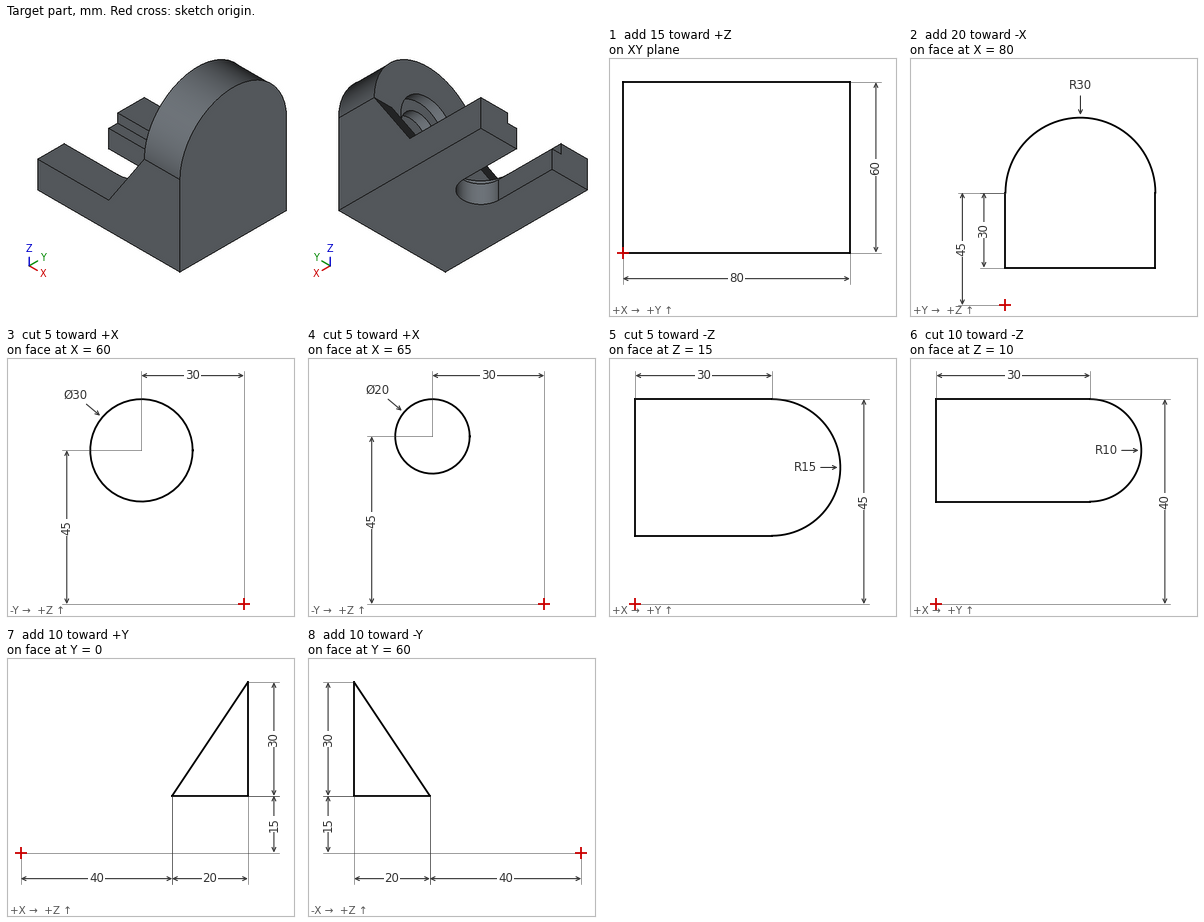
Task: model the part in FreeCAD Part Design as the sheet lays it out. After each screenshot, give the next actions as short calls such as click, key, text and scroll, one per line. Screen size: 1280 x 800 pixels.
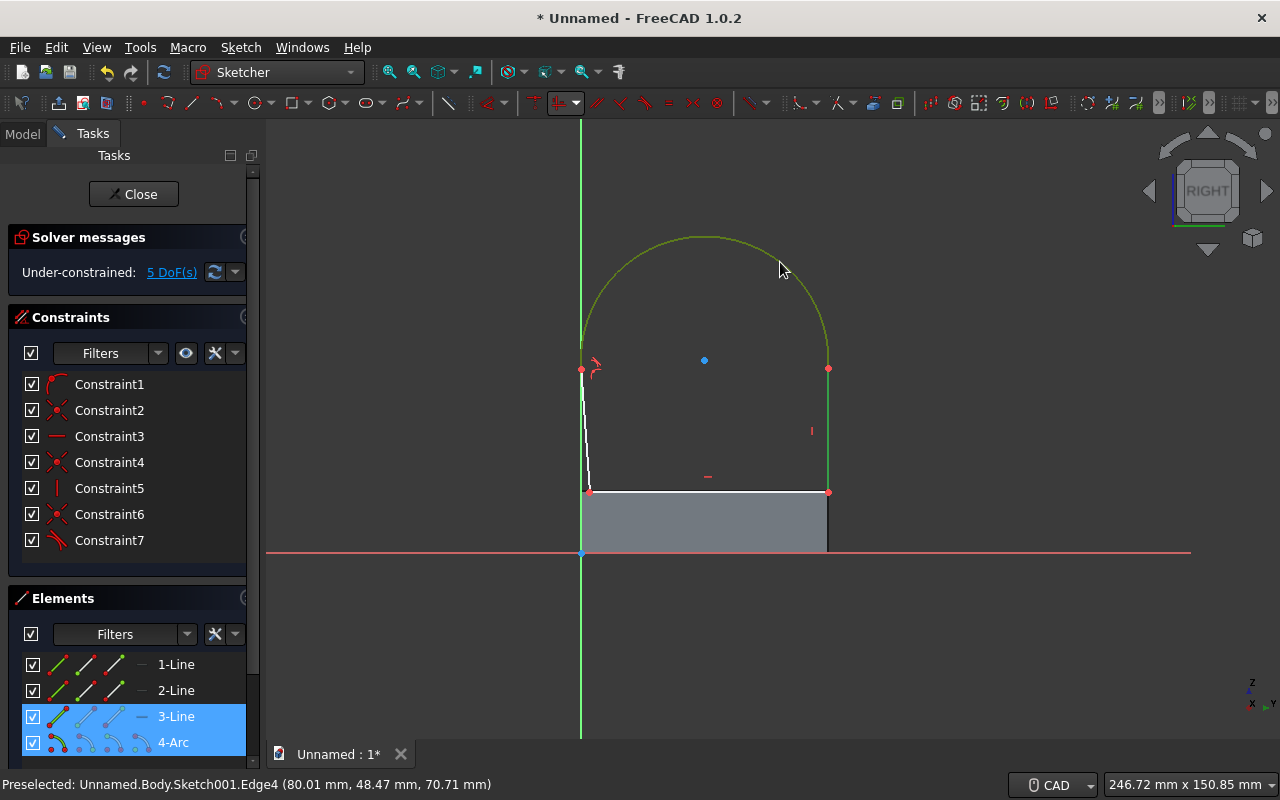
click(646, 104)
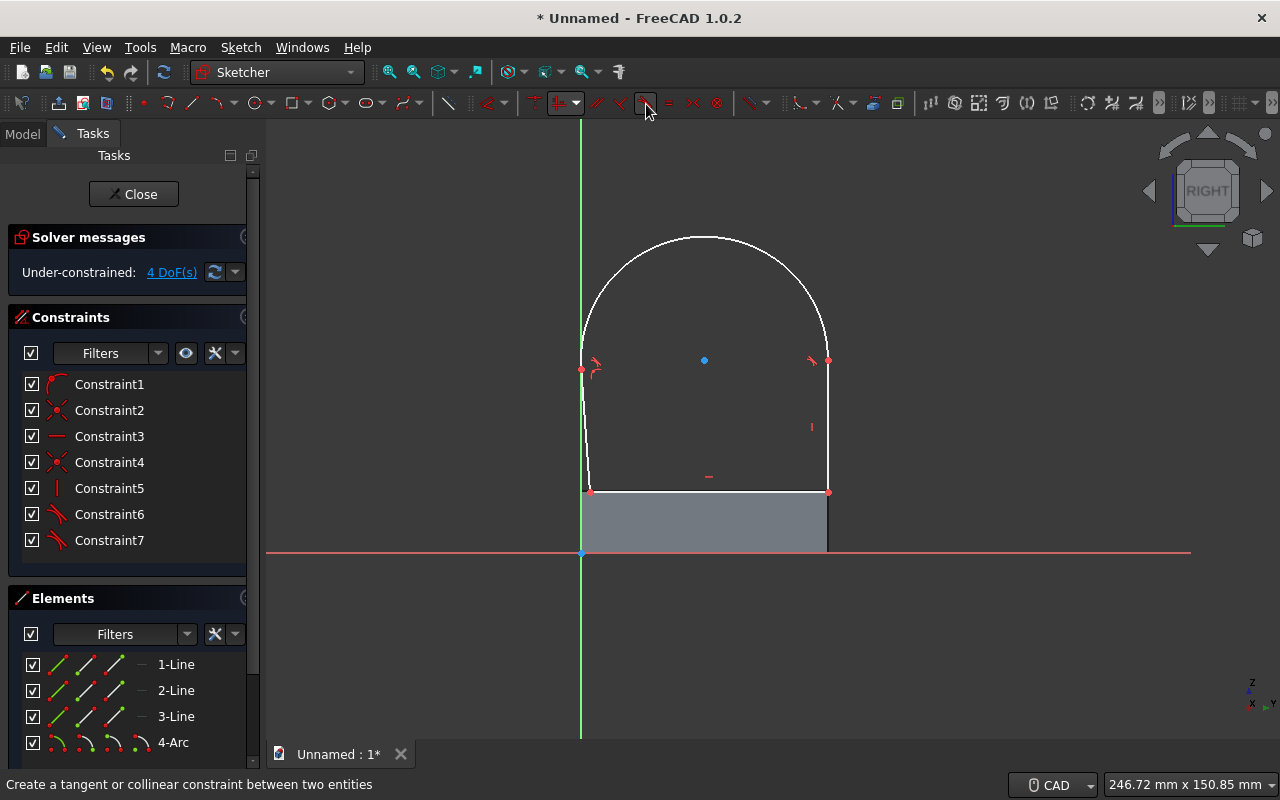
click(584, 406)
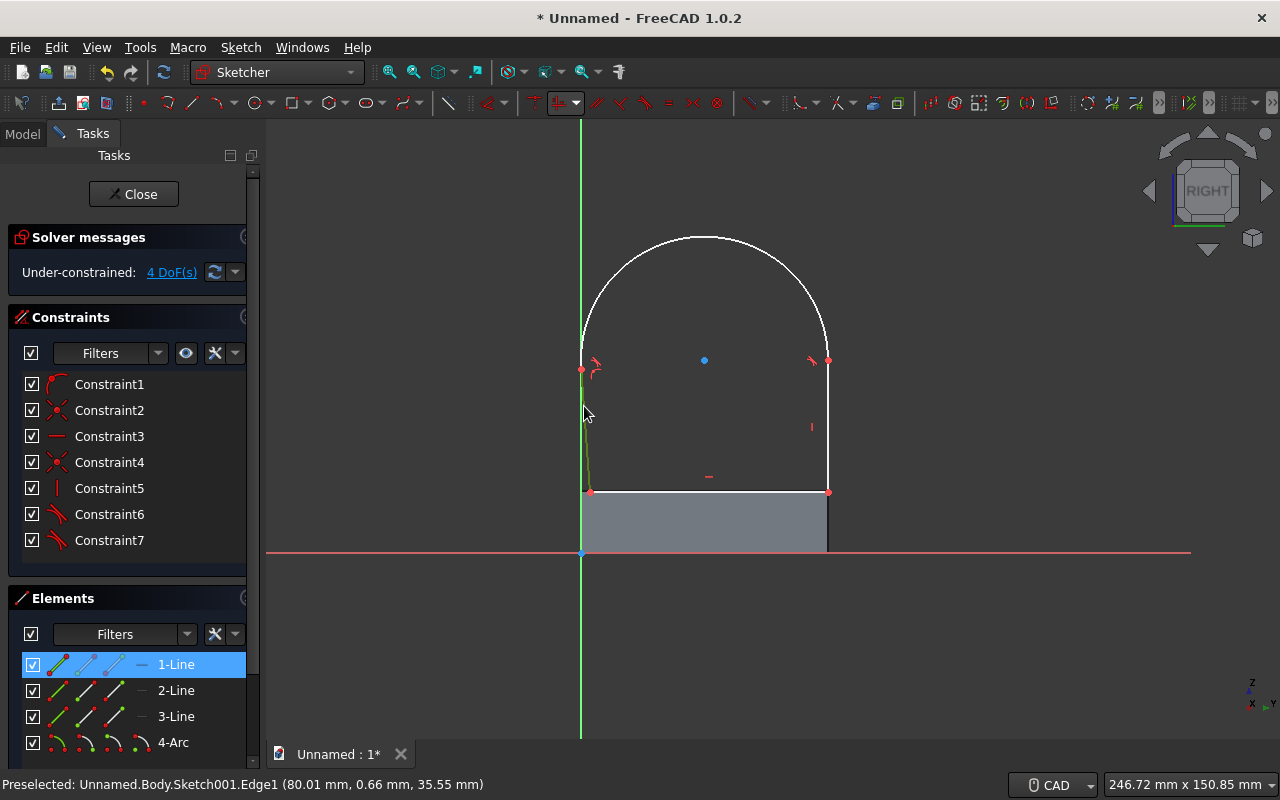
key(v)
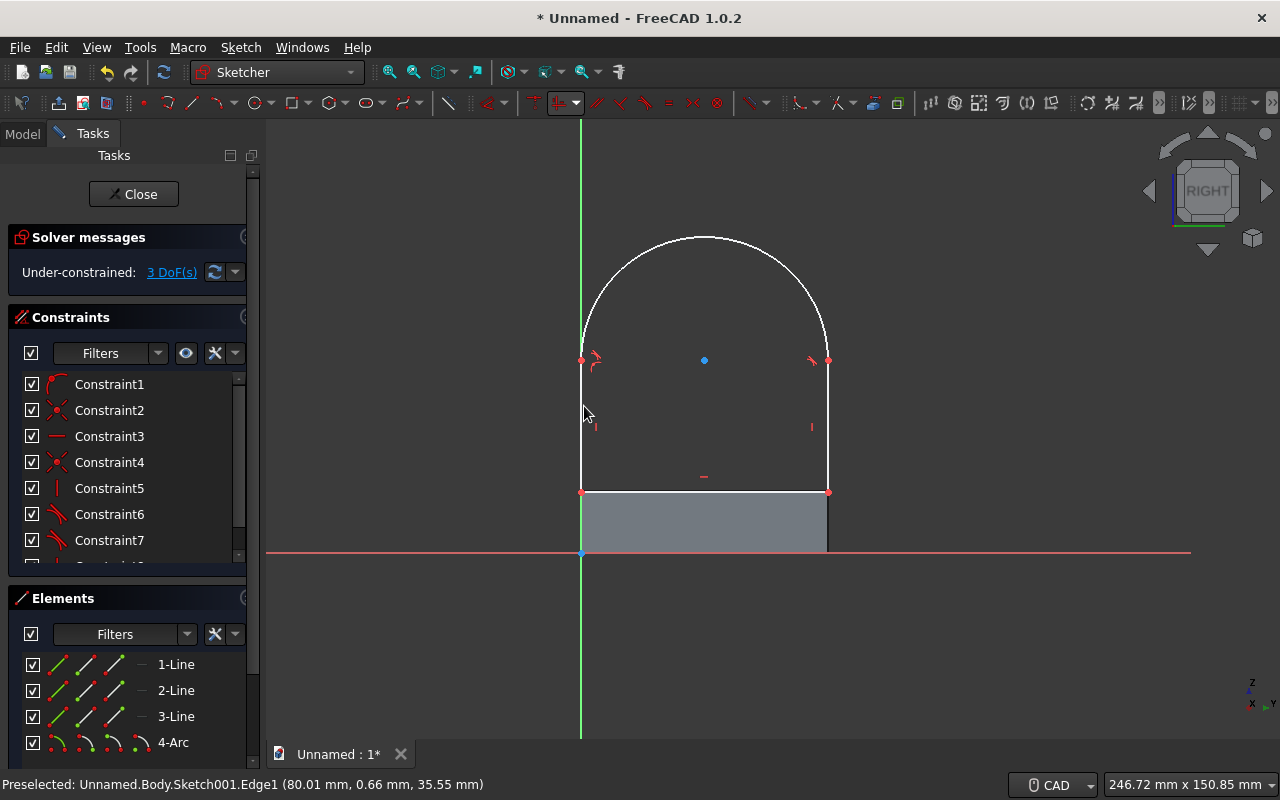
click(488, 104)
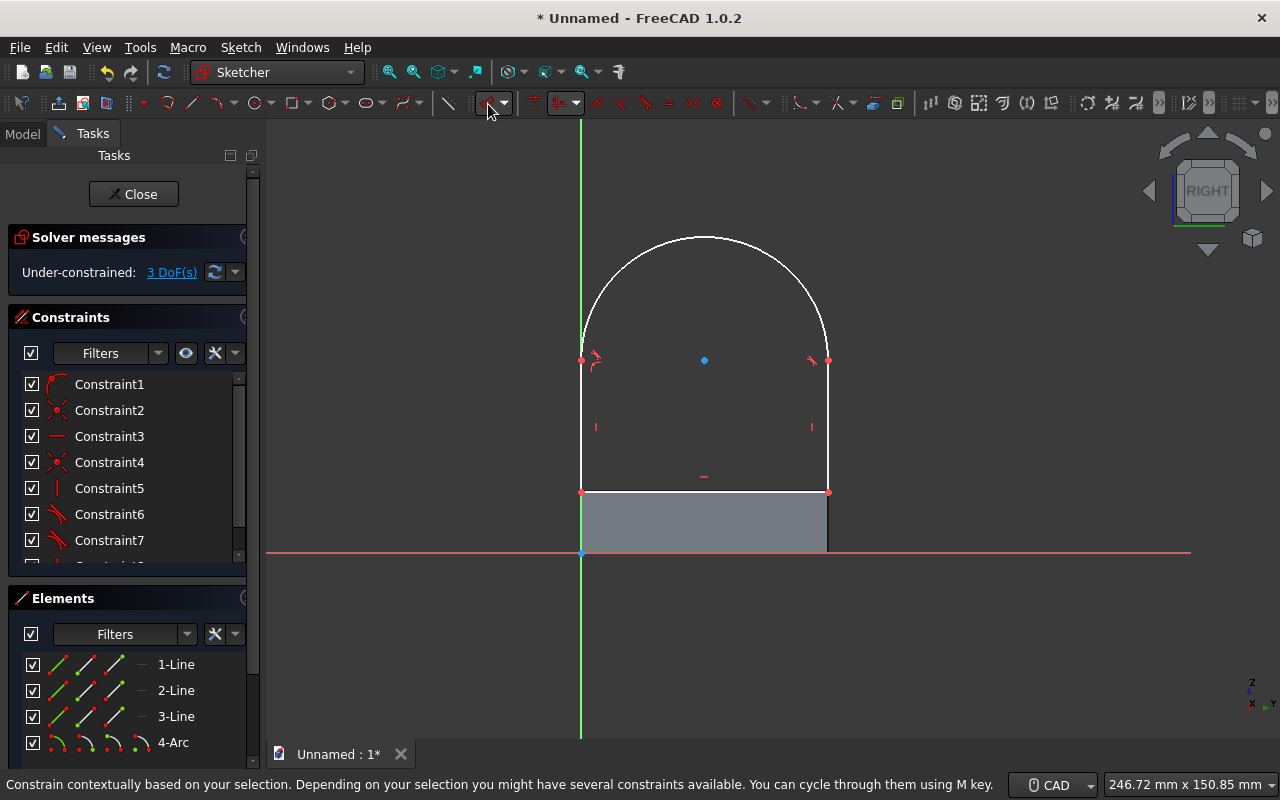
click(777, 261)
click(796, 235)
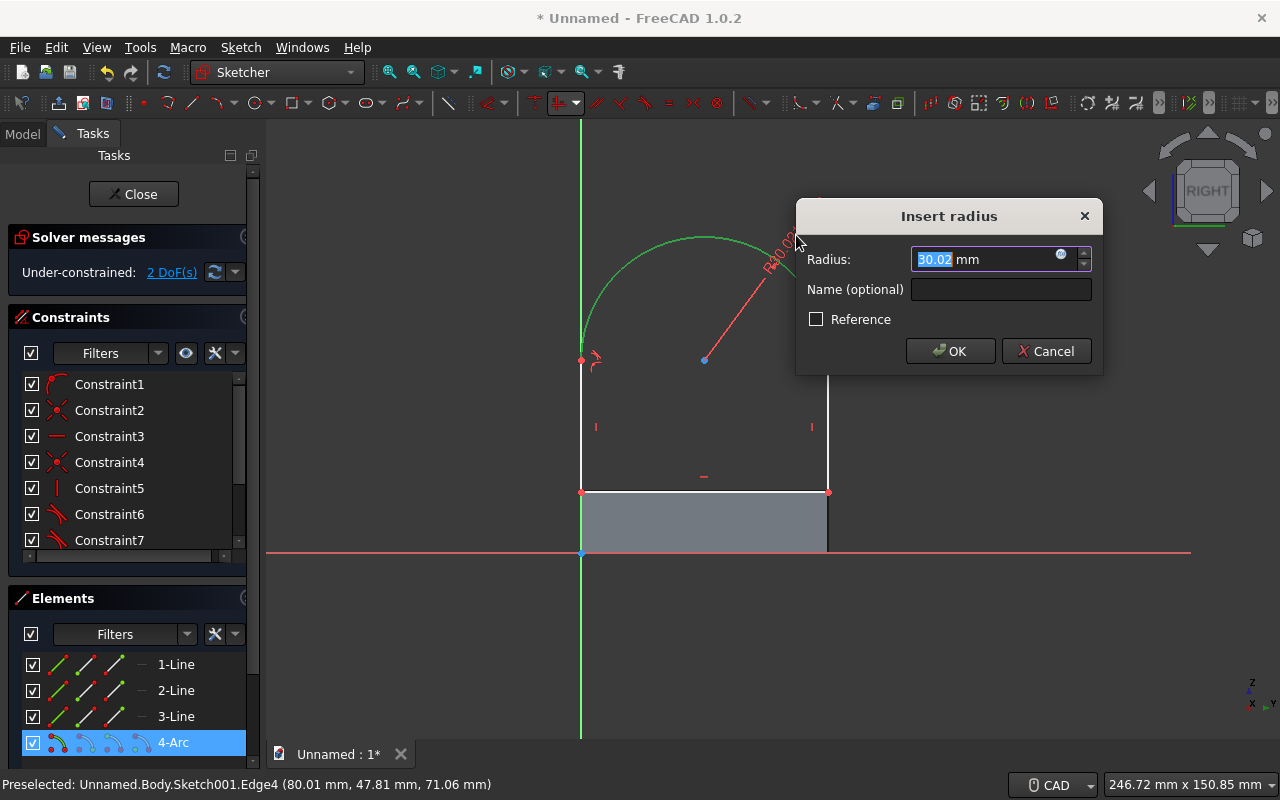
text(30)
key(Return)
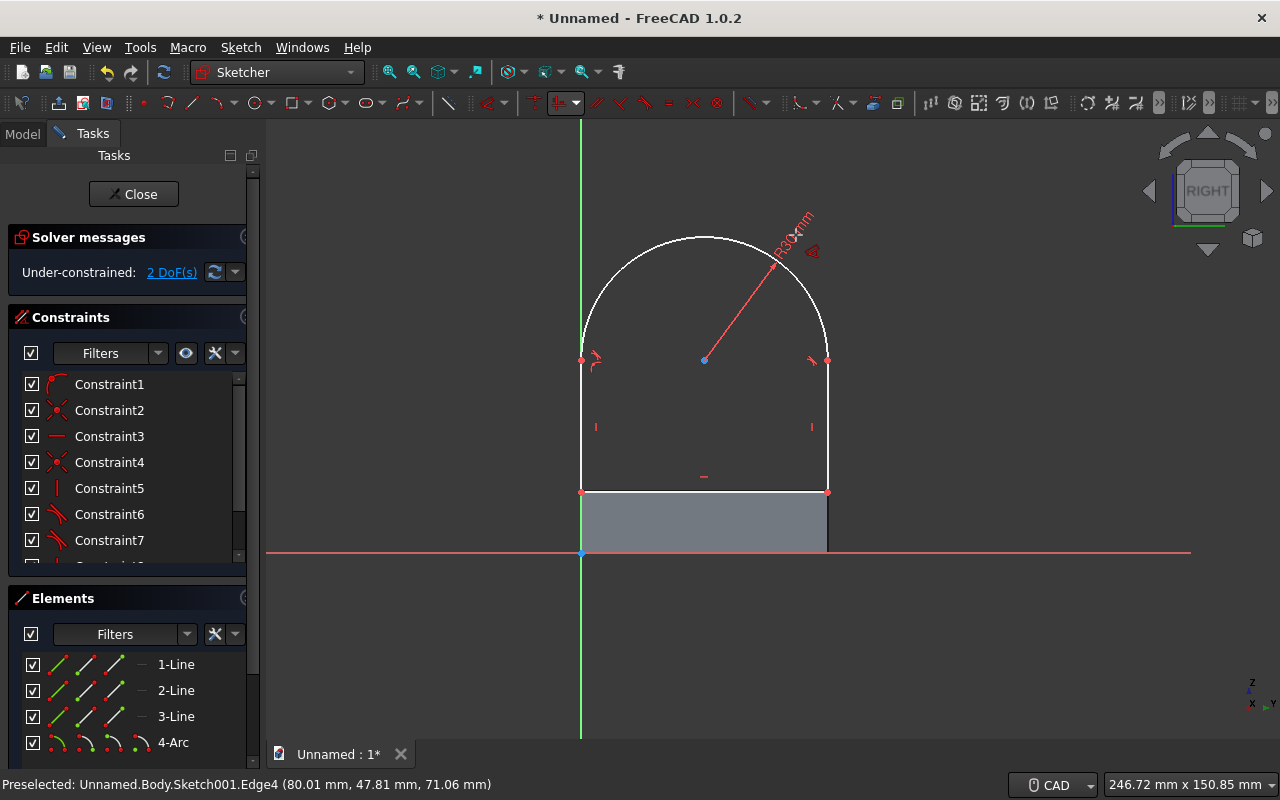
click(581, 400)
click(547, 426)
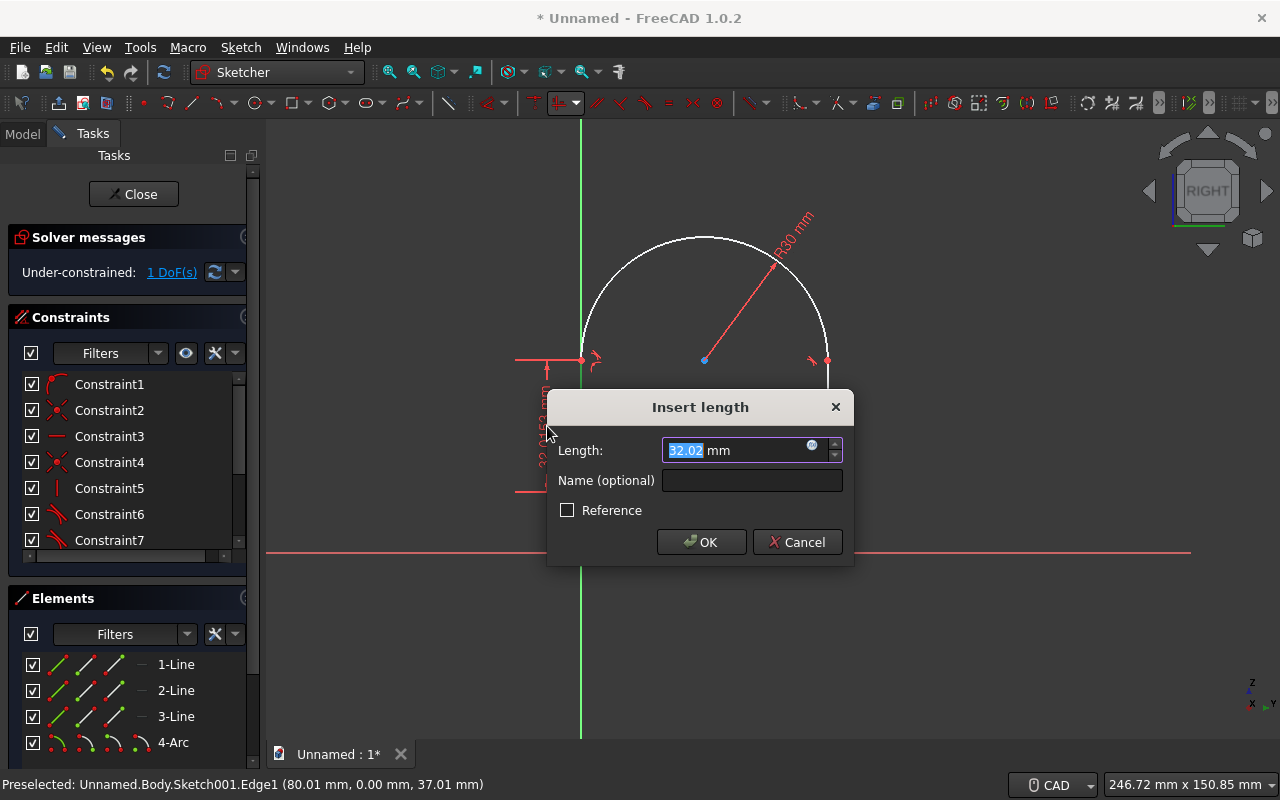
text(30)
key(Return)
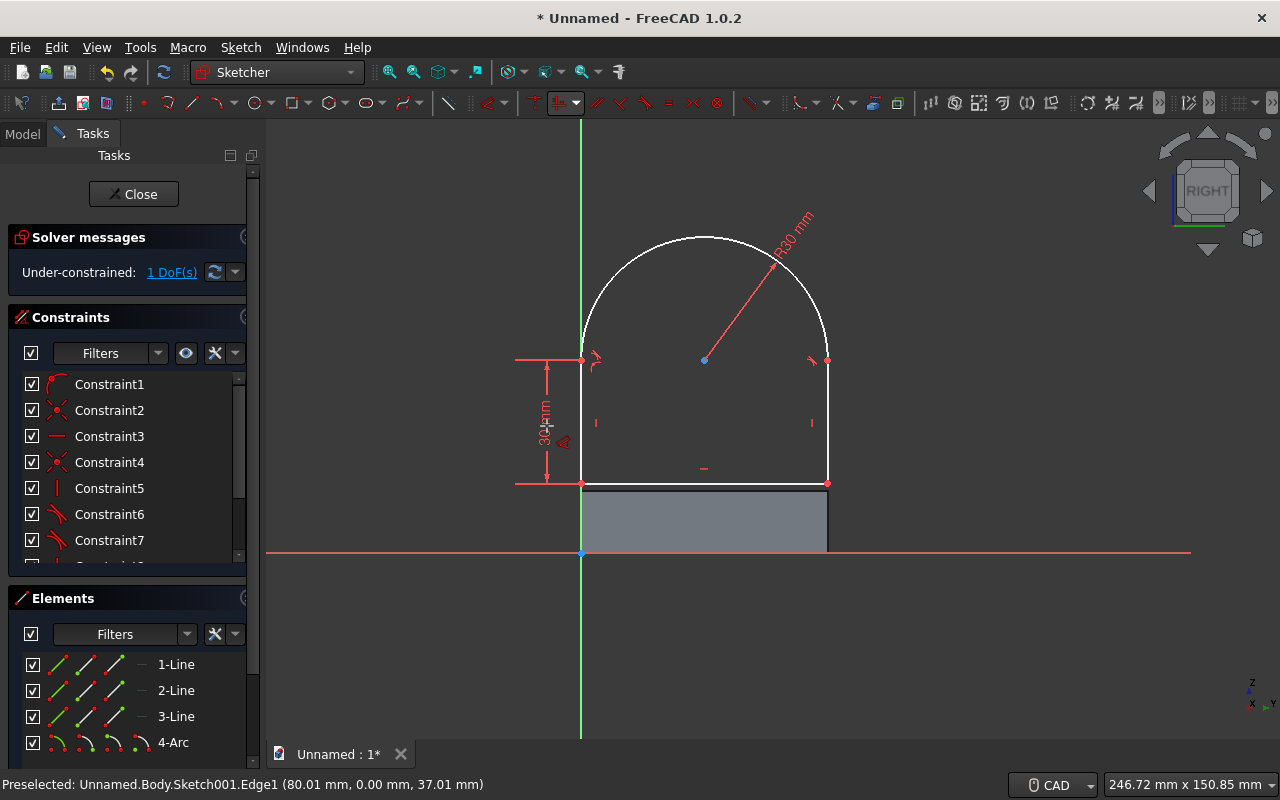
click(581, 360)
click(547, 457)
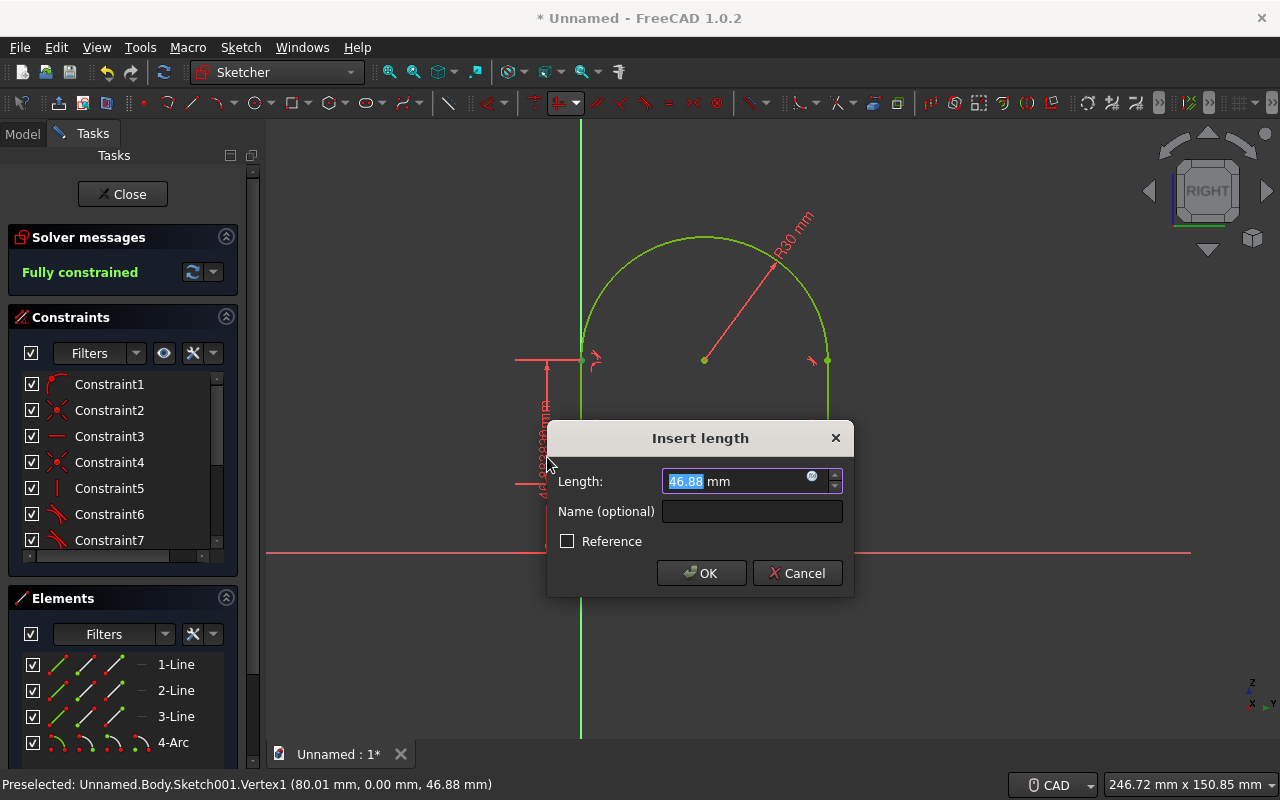
text(45)
key(Return)
key(Escape)